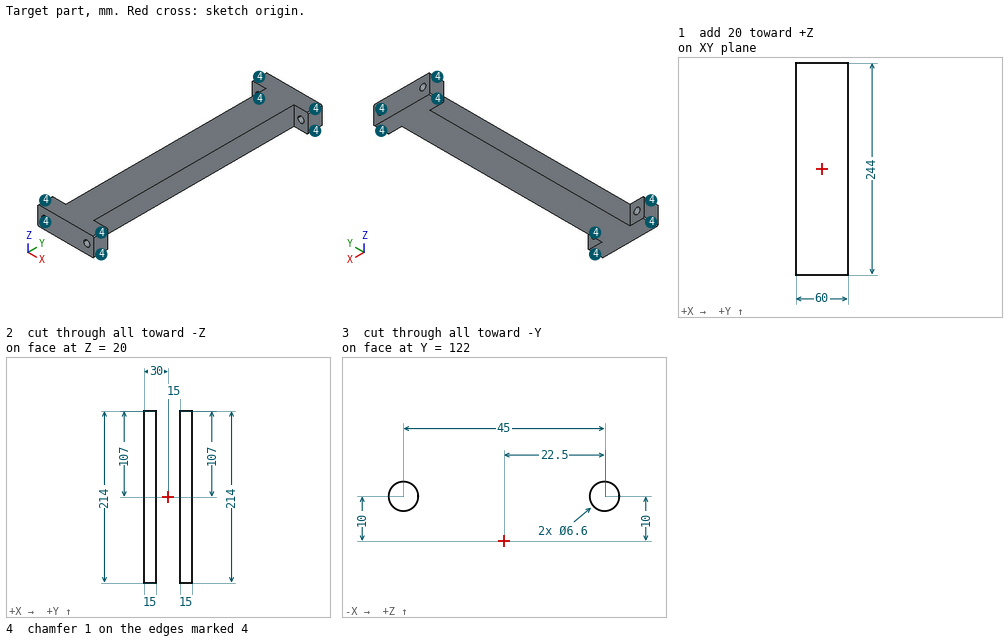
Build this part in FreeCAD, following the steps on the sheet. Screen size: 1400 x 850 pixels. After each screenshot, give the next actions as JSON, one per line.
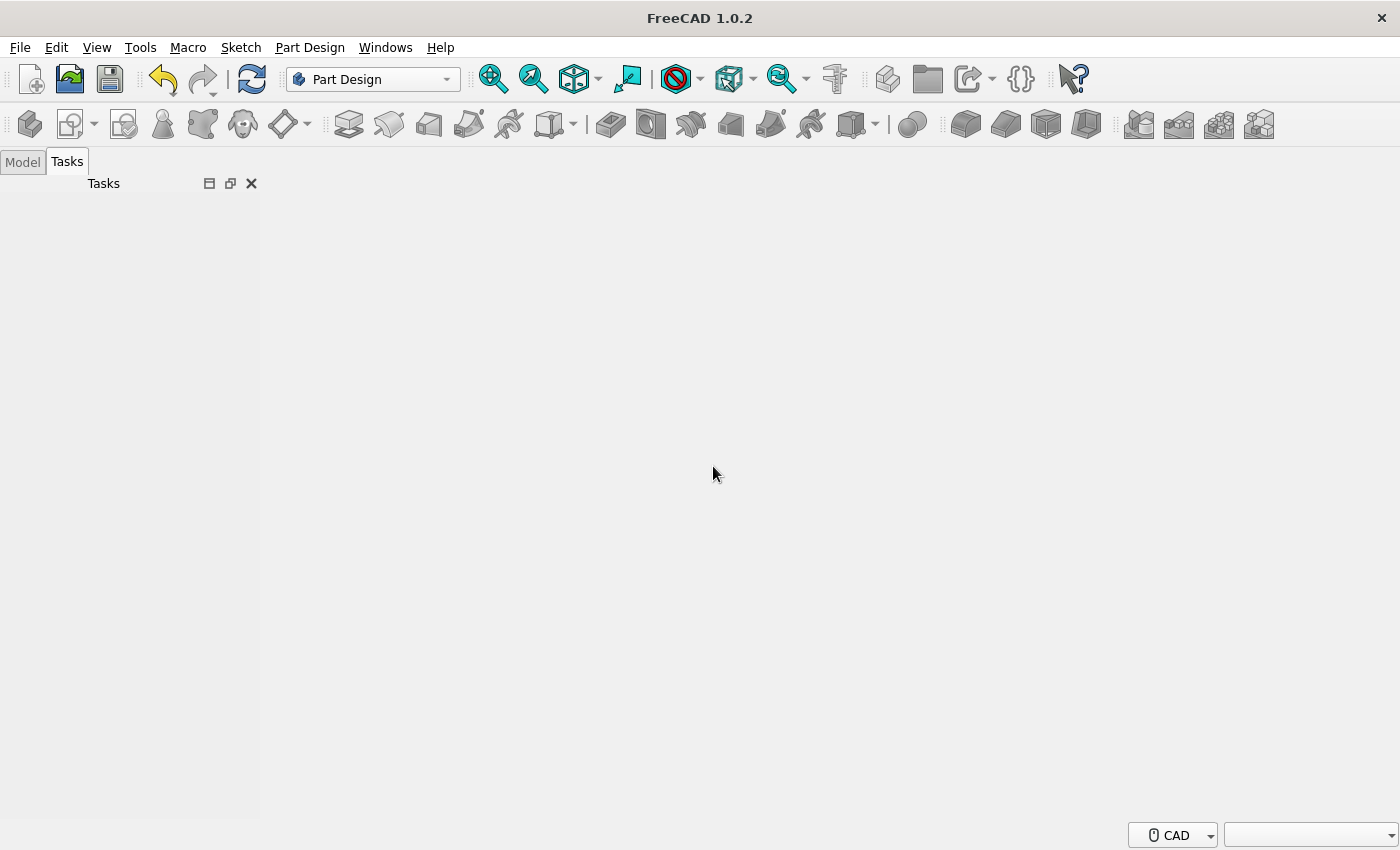
{"action": "left_click", "coordinate": [30, 80]}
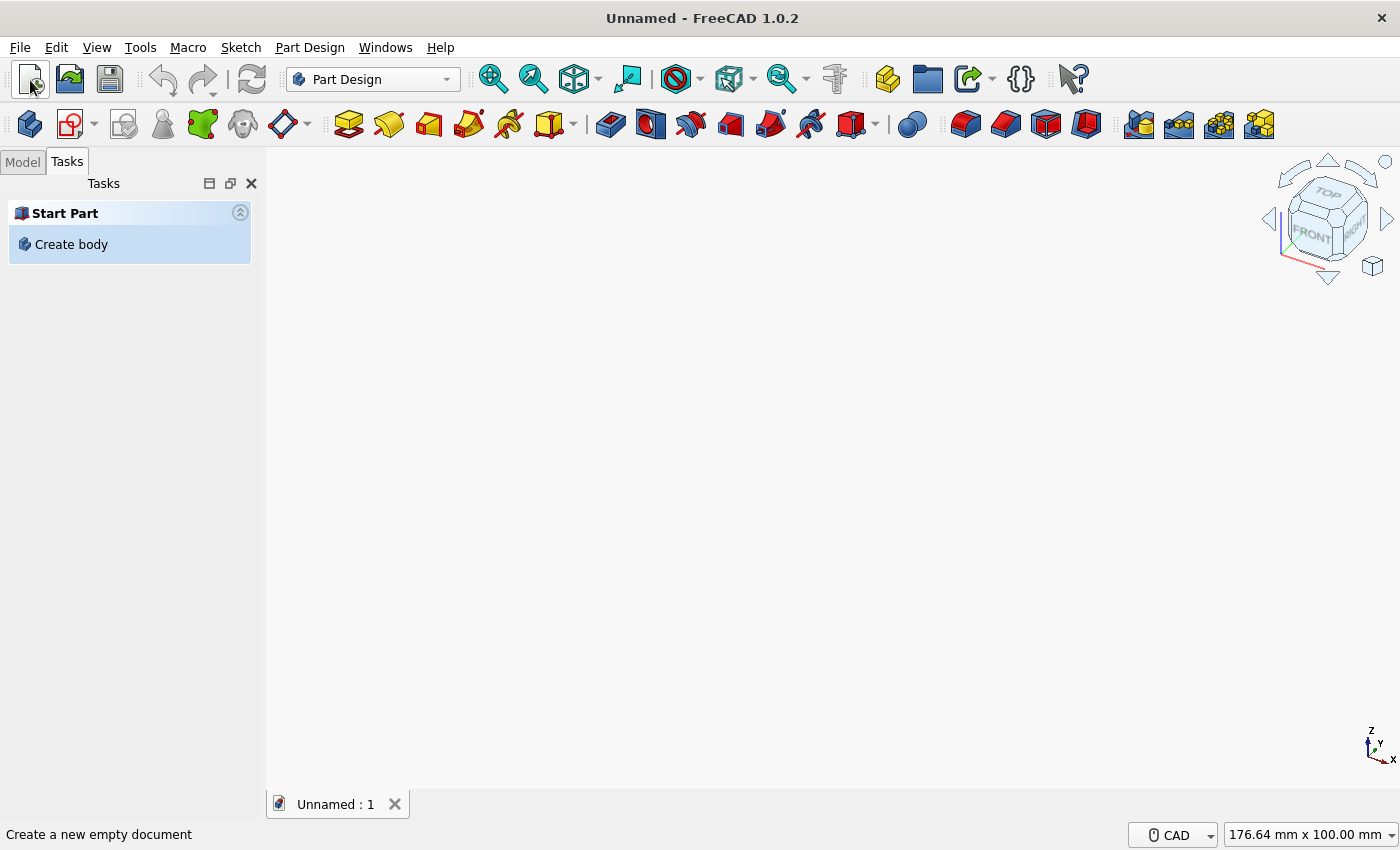
{"action": "left_click", "coordinate": [70, 124]}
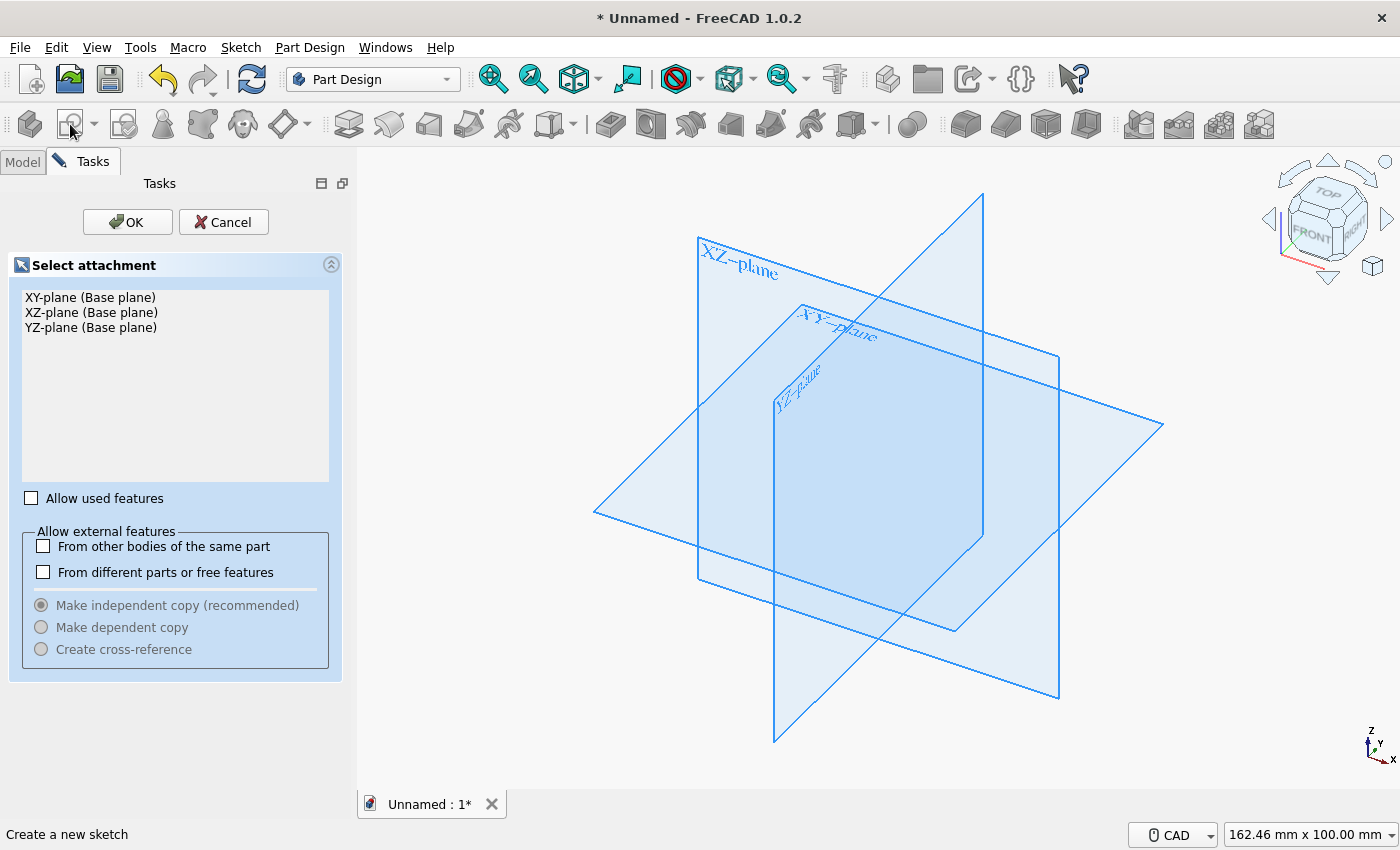
{"action": "left_click", "coordinate": [82, 298]}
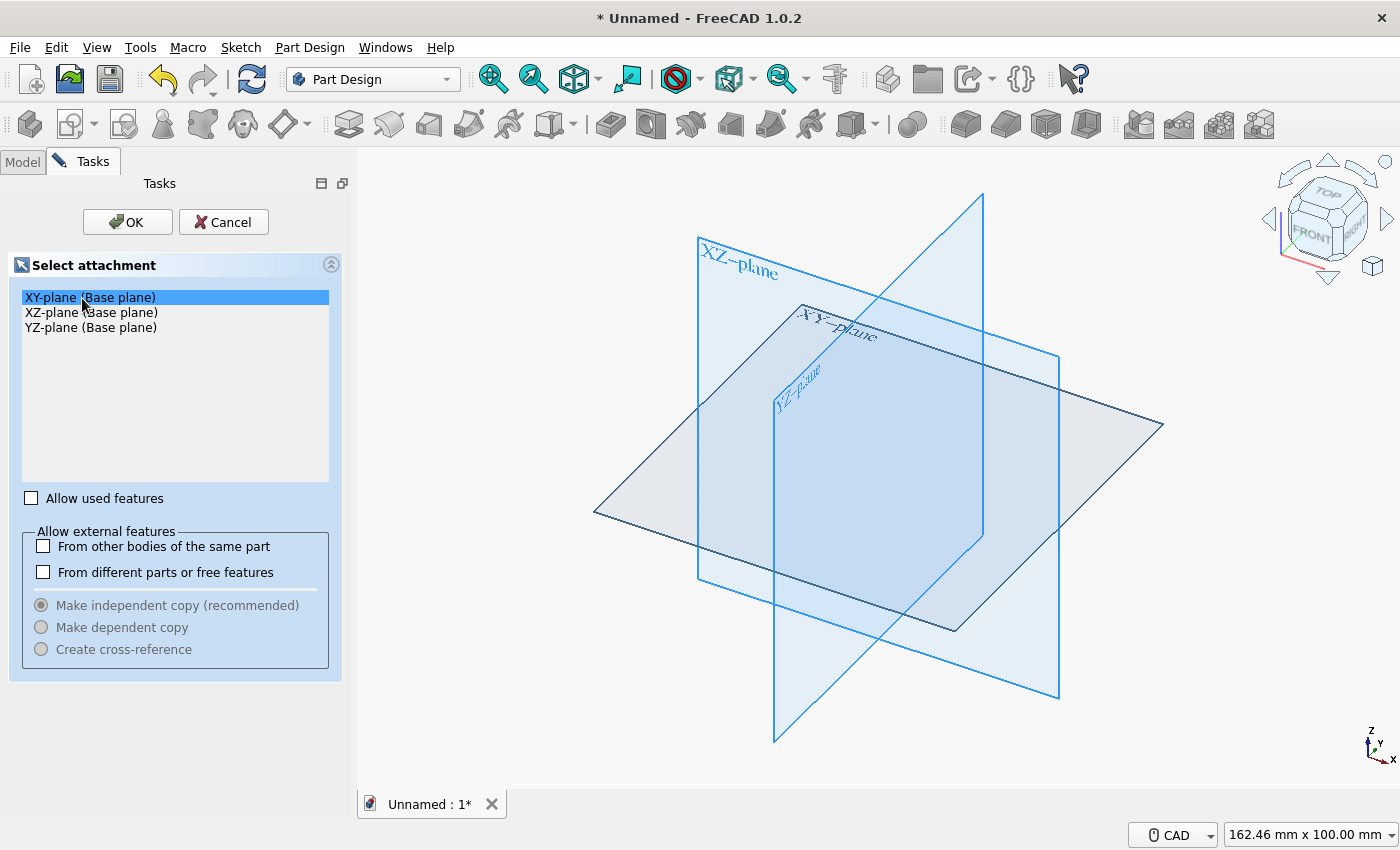
{"action": "left_click", "coordinate": [128, 222]}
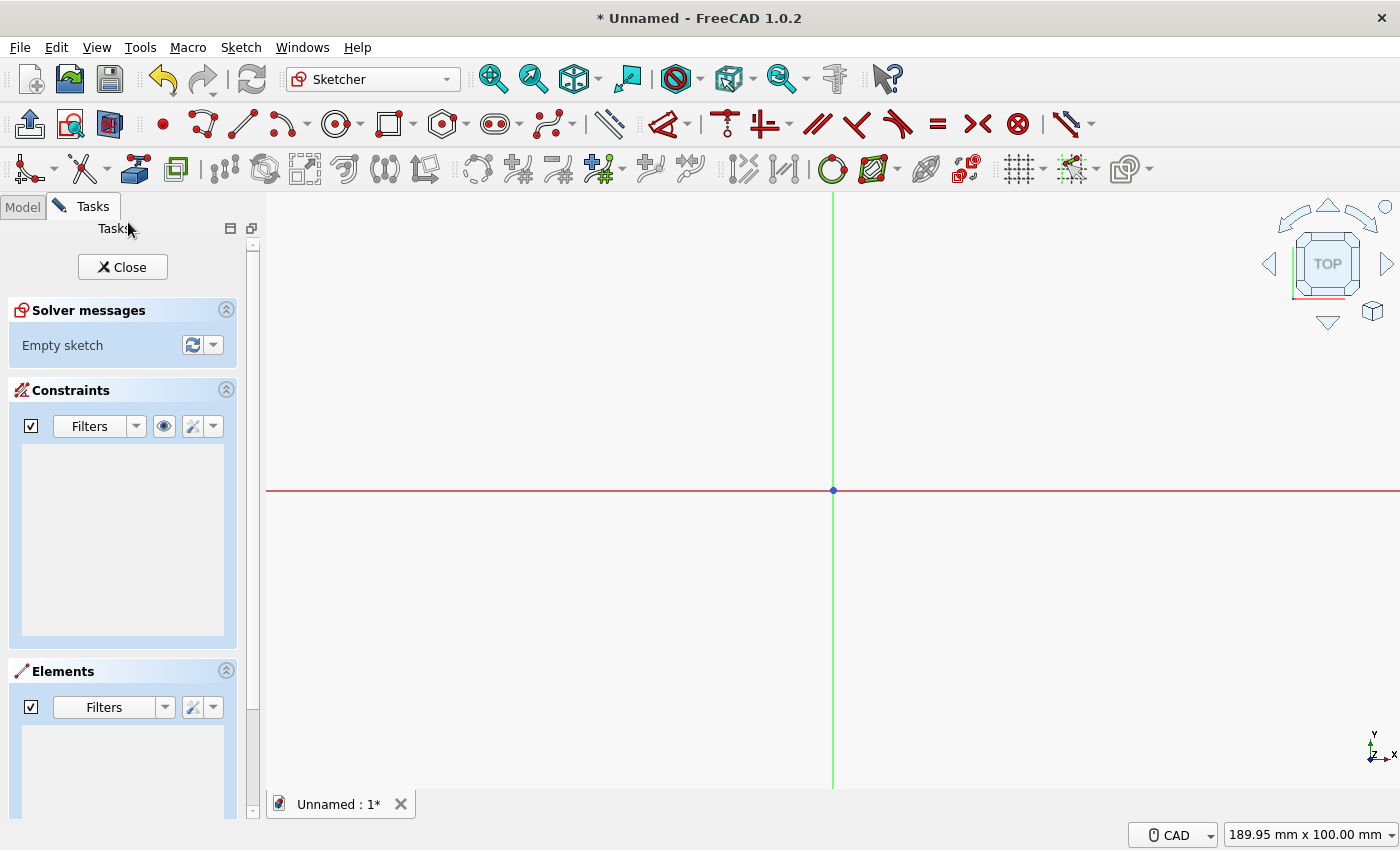
{"action": "scroll", "coordinate": [742, 490], "scroll_direction": "down", "scroll_amount": 7}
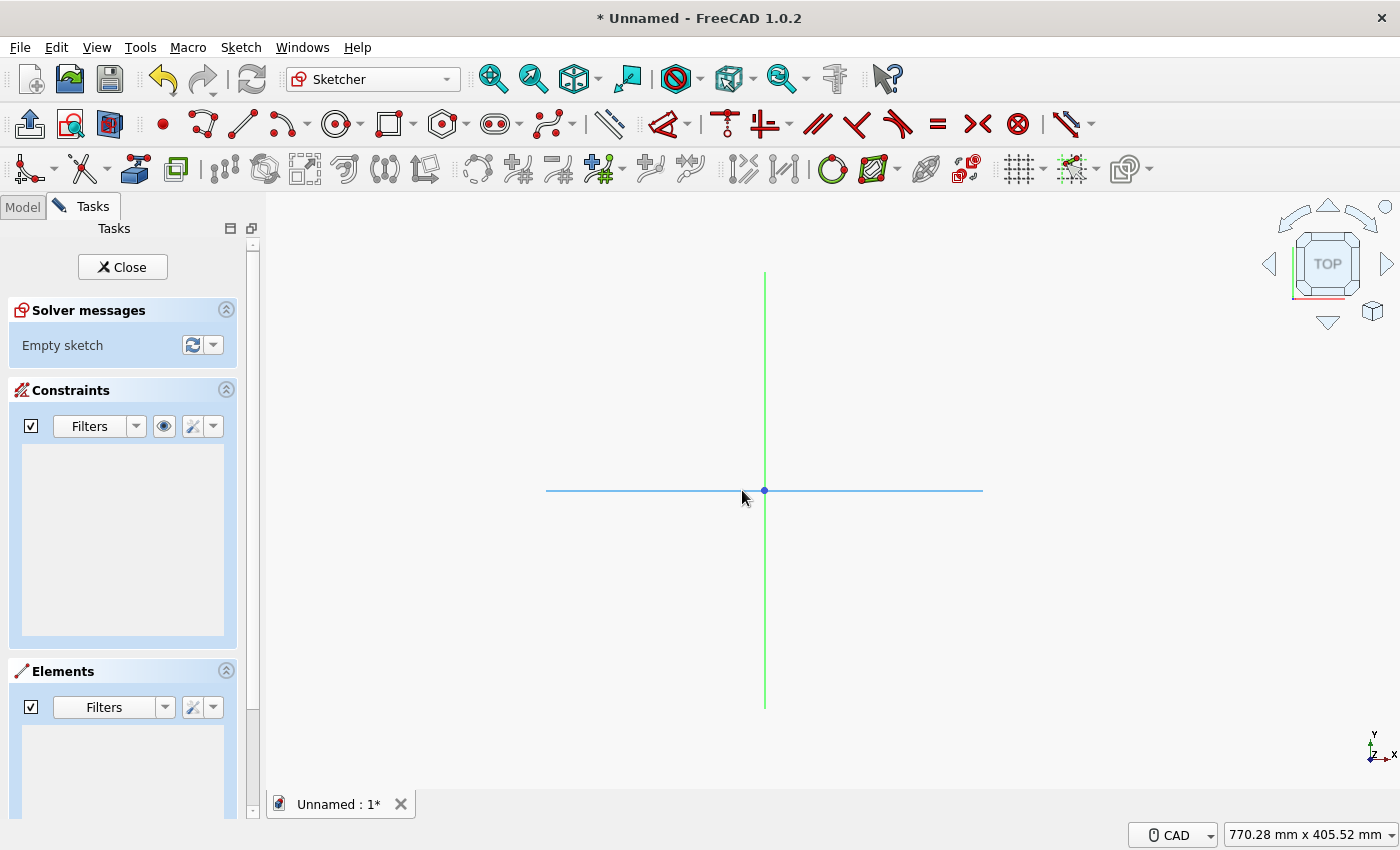
{"action": "left_click", "coordinate": [416, 124]}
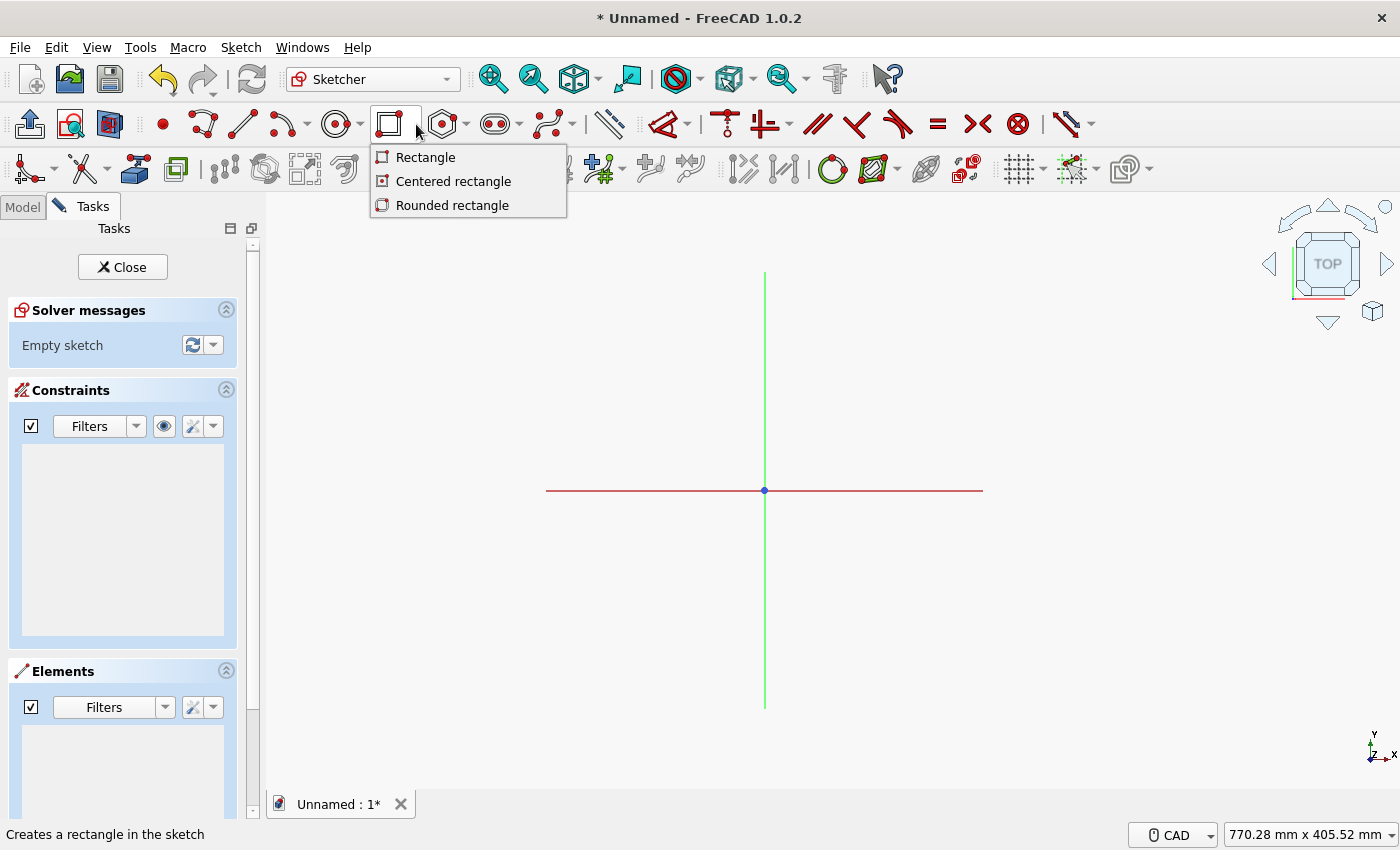
{"action": "left_click", "coordinate": [468, 181]}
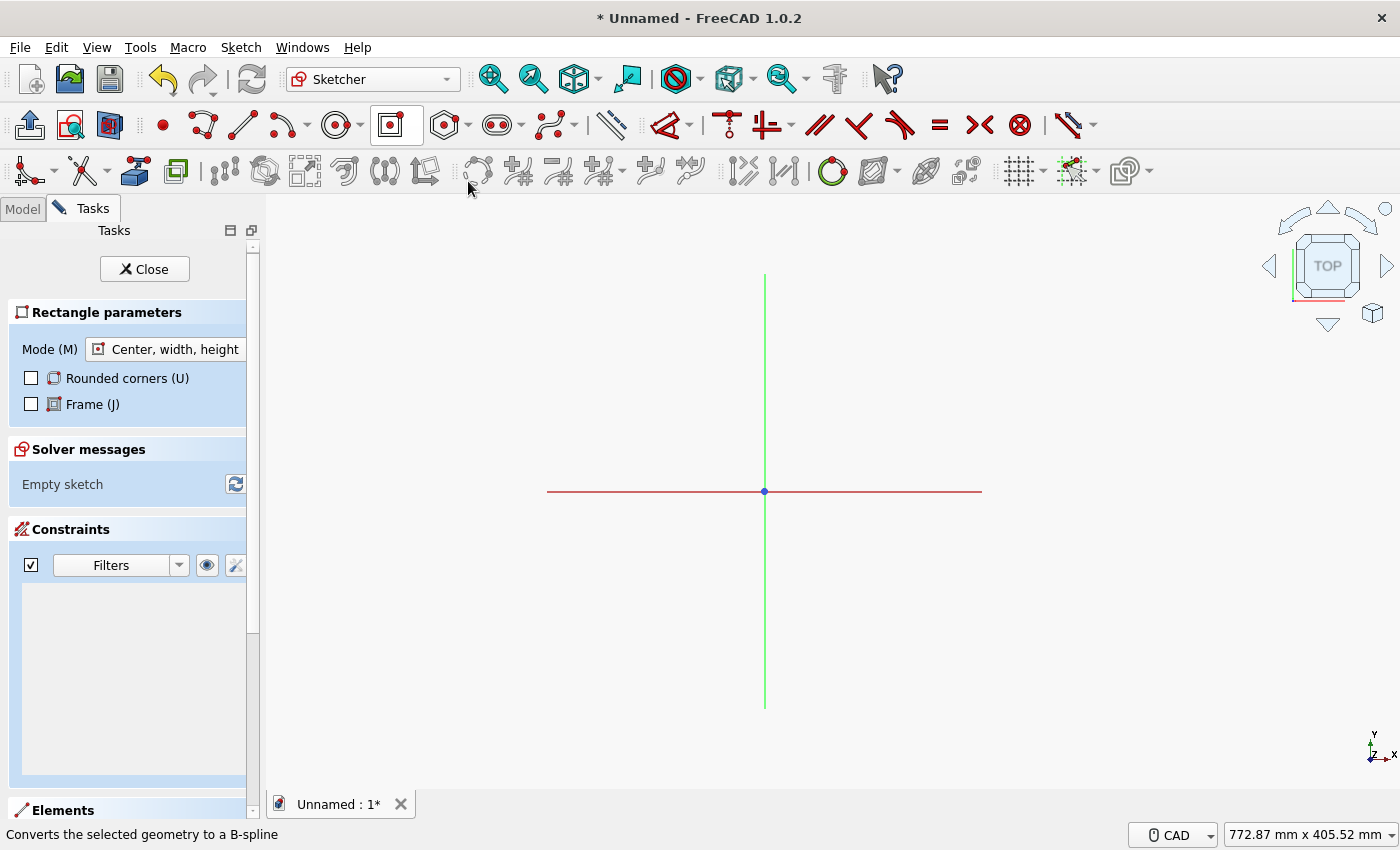
{"action": "left_click", "coordinate": [765, 492]}
{"action": "mouse_move", "coordinate": [809, 312]}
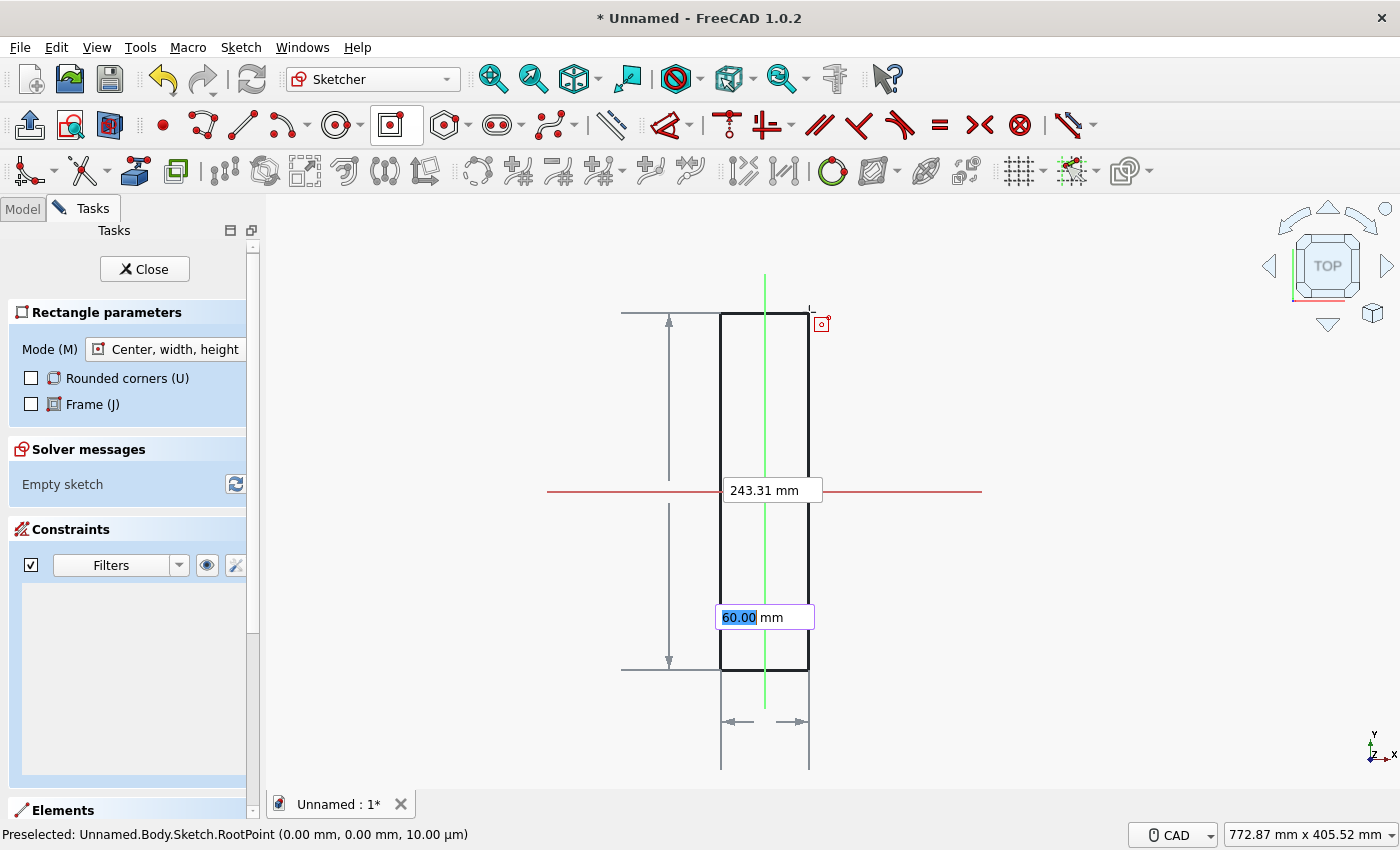
{"action": "type", "text": "60"}
{"action": "key", "text": "Tab"}
{"action": "type", "text": "244"}
{"action": "key", "text": "Return"}
{"action": "key", "text": "Escape"}